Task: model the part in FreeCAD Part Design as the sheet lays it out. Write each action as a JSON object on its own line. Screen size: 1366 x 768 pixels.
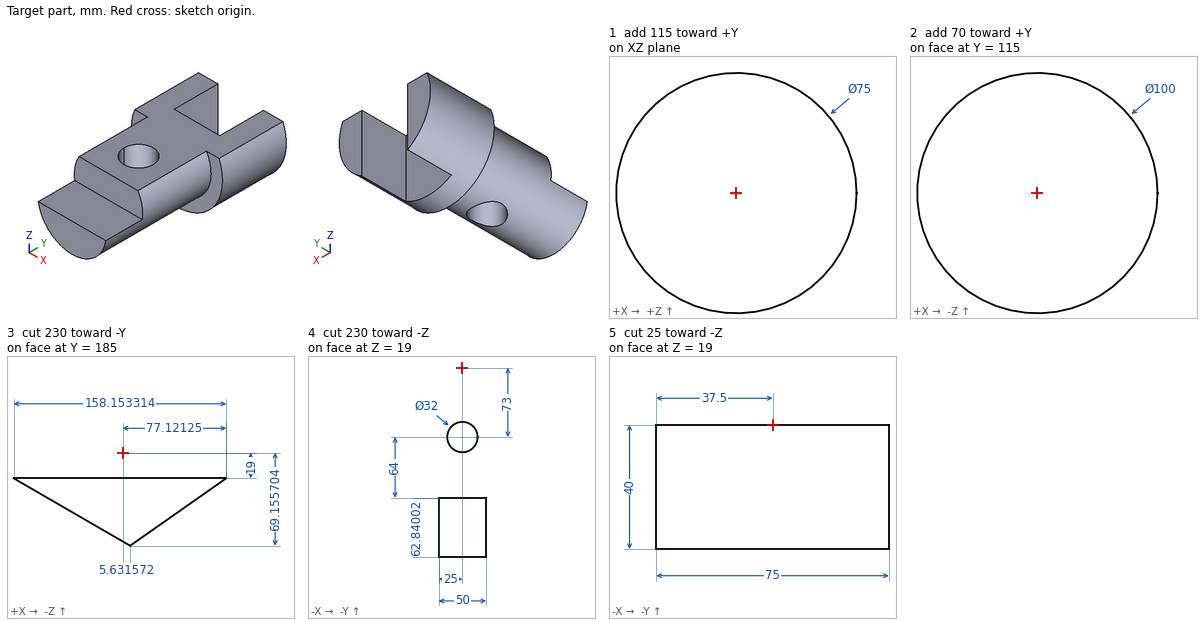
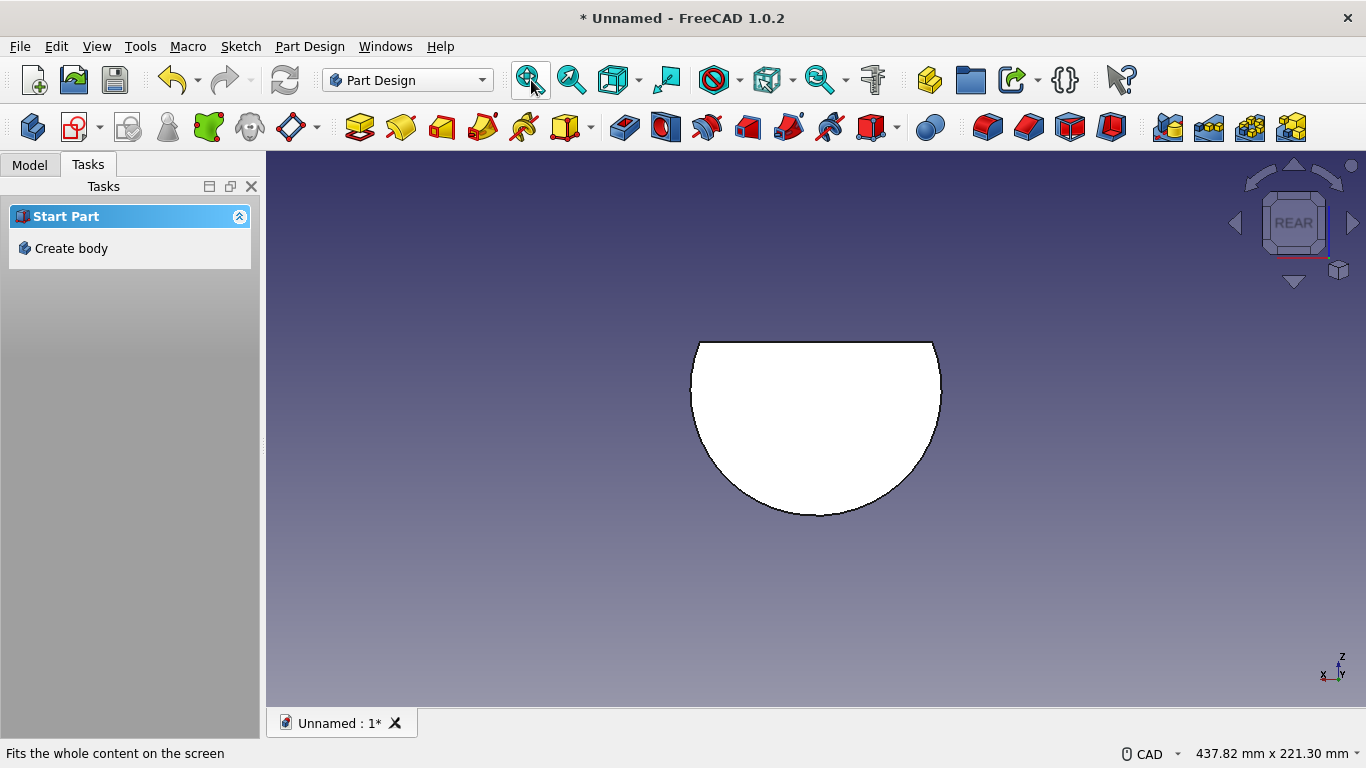
{"action": "key", "text": "0"}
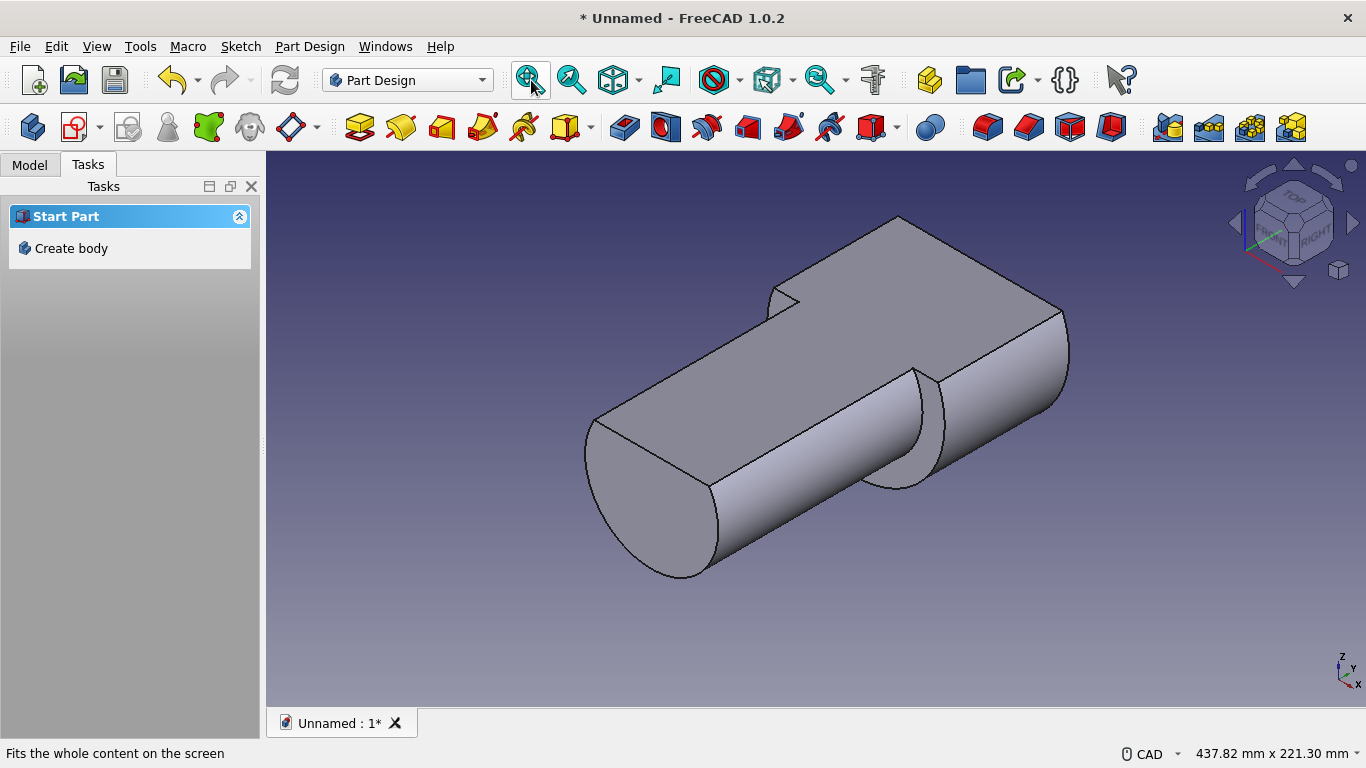
{"action": "left_click", "coordinate": [910, 303]}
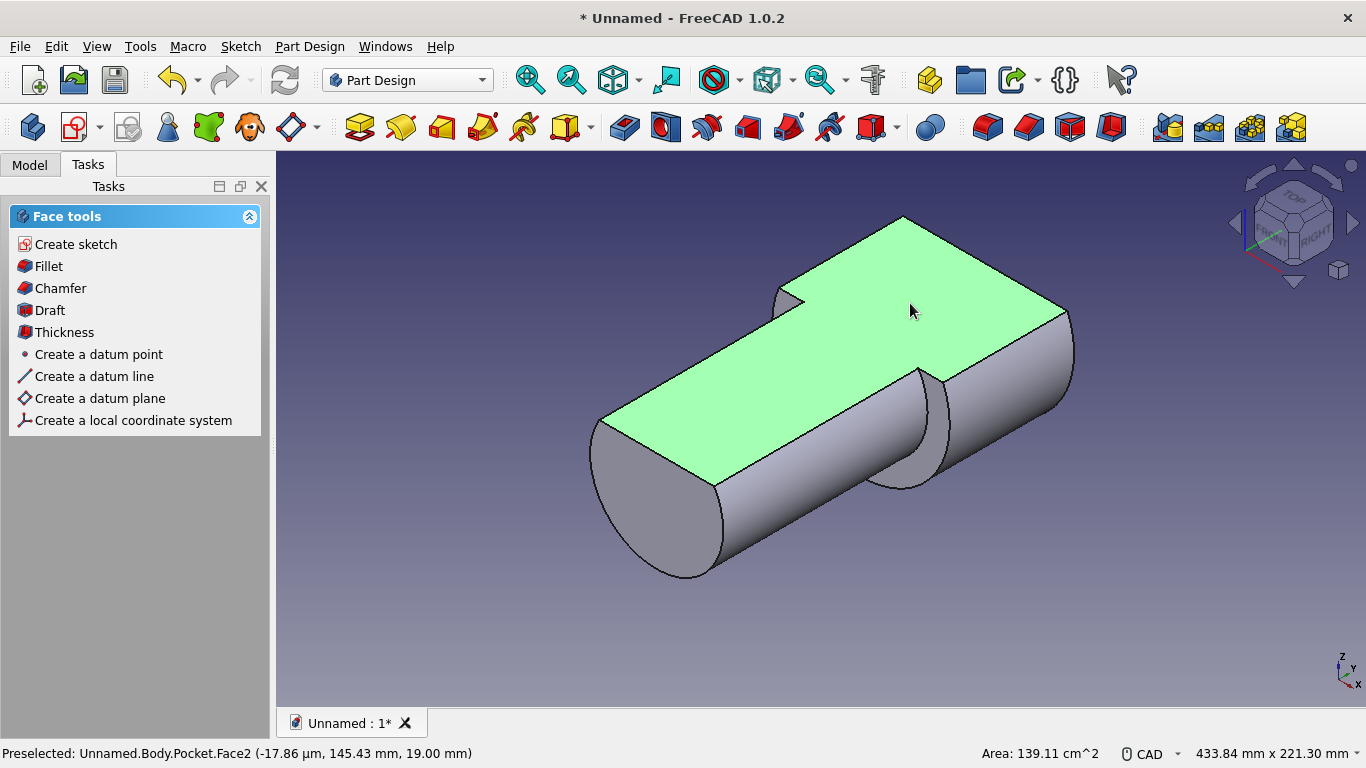
{"action": "left_click", "coordinate": [74, 128]}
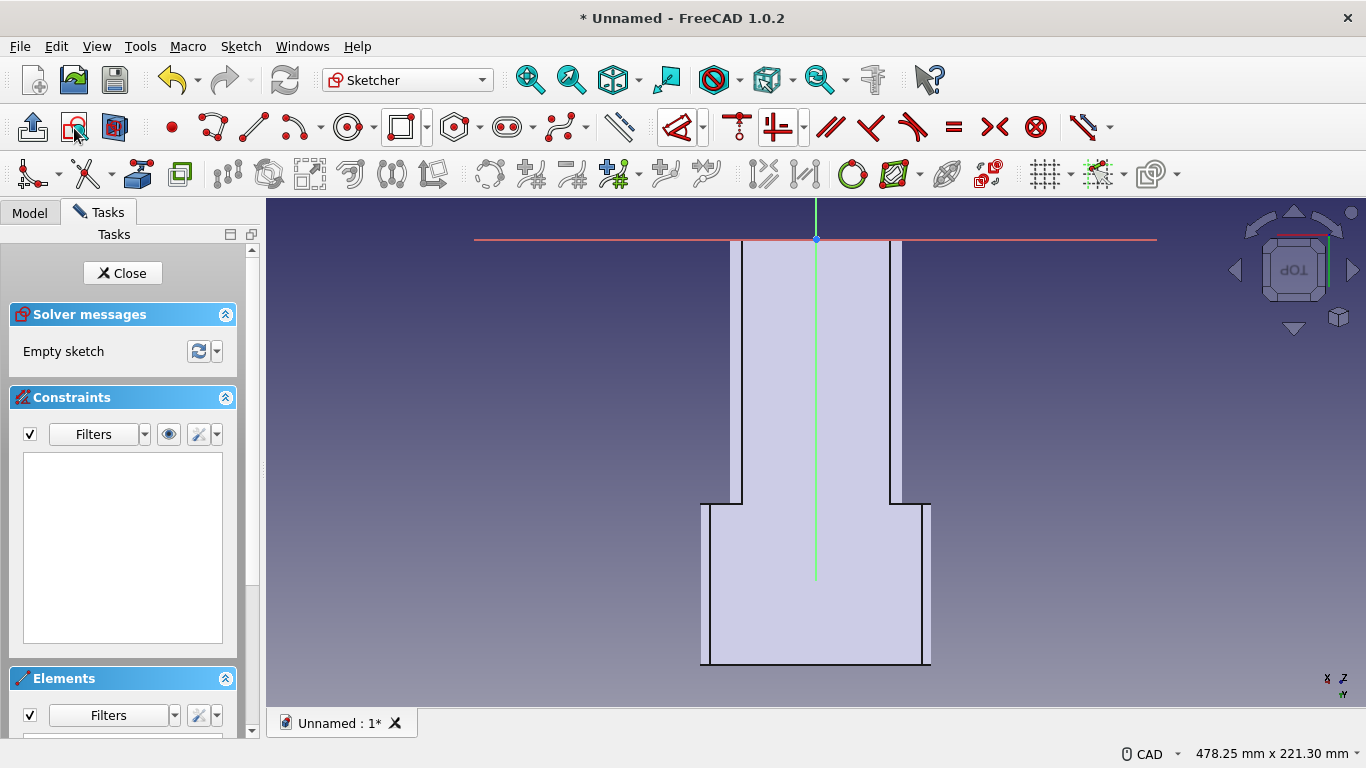
{"action": "scroll", "coordinate": [608, 418], "scroll_direction": "down", "scroll_amount": 2}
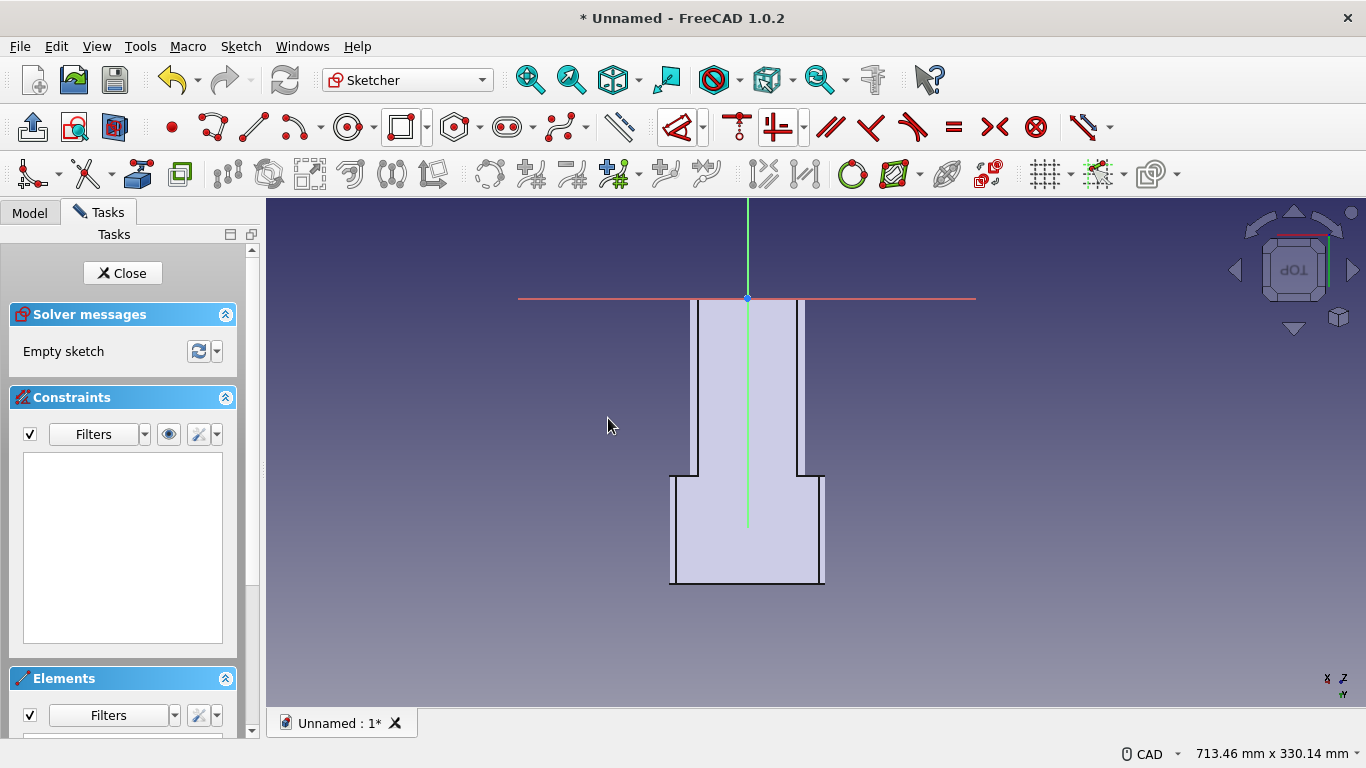
{"action": "left_click", "coordinate": [400, 128]}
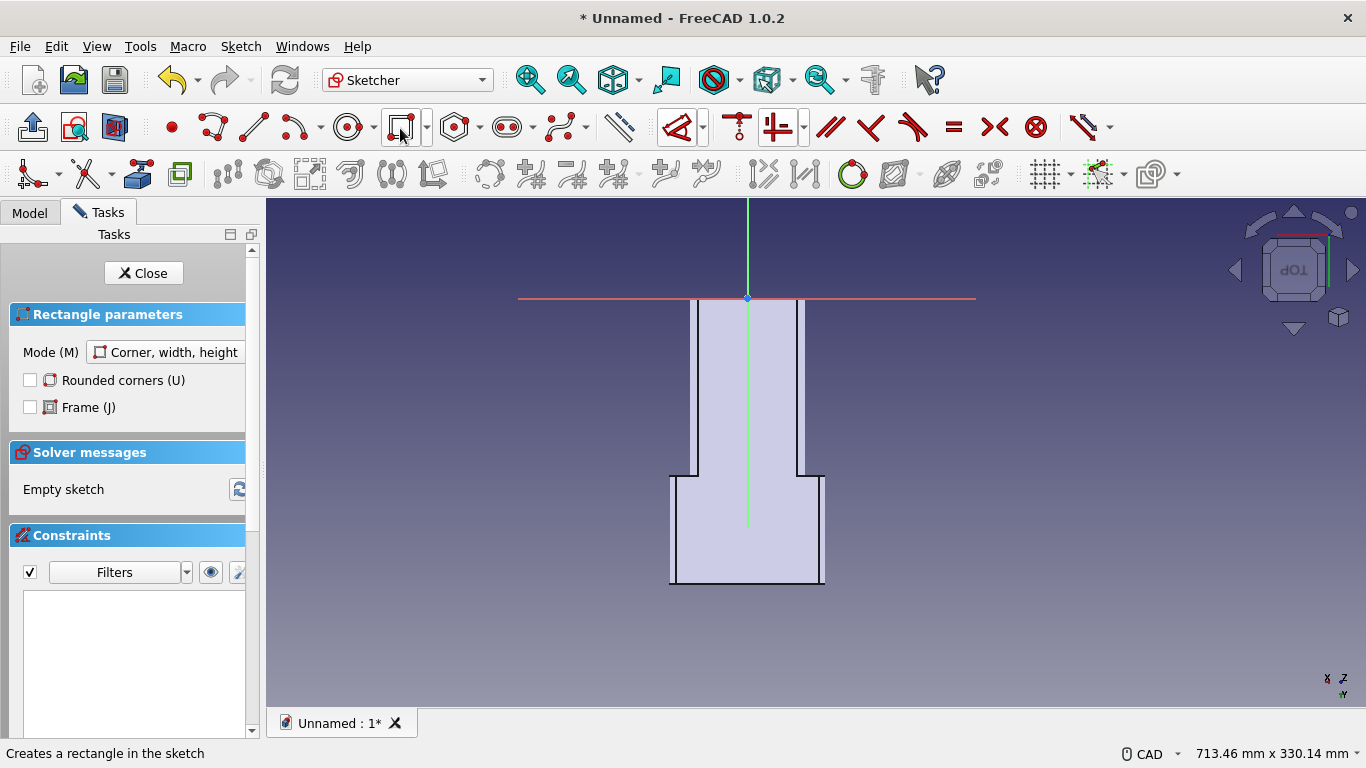
{"action": "left_click", "coordinate": [709, 510]}
{"action": "left_click", "coordinate": [786, 607]}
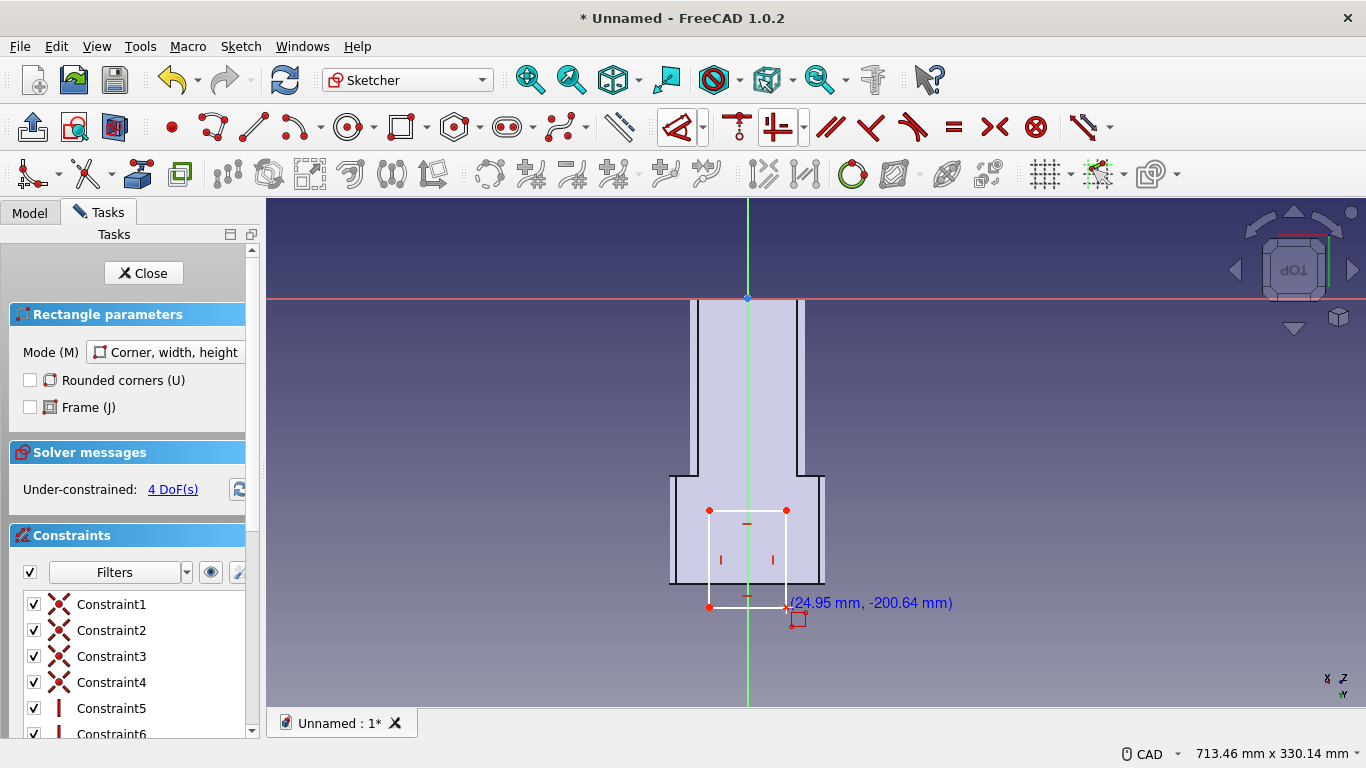
{"action": "left_click", "coordinate": [348, 128]}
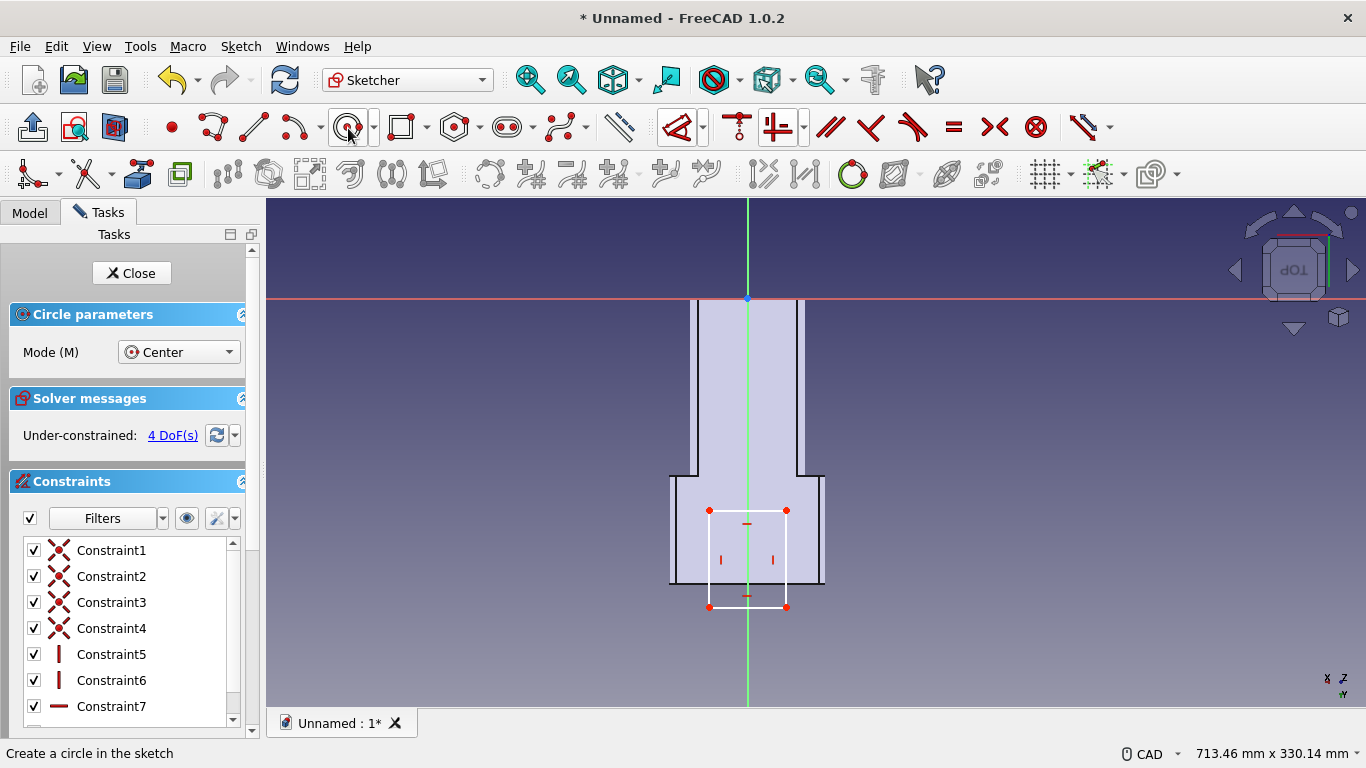
{"action": "left_click", "coordinate": [748, 411]}
{"action": "left_click", "coordinate": [765, 394]}
{"action": "key", "text": "Escape"}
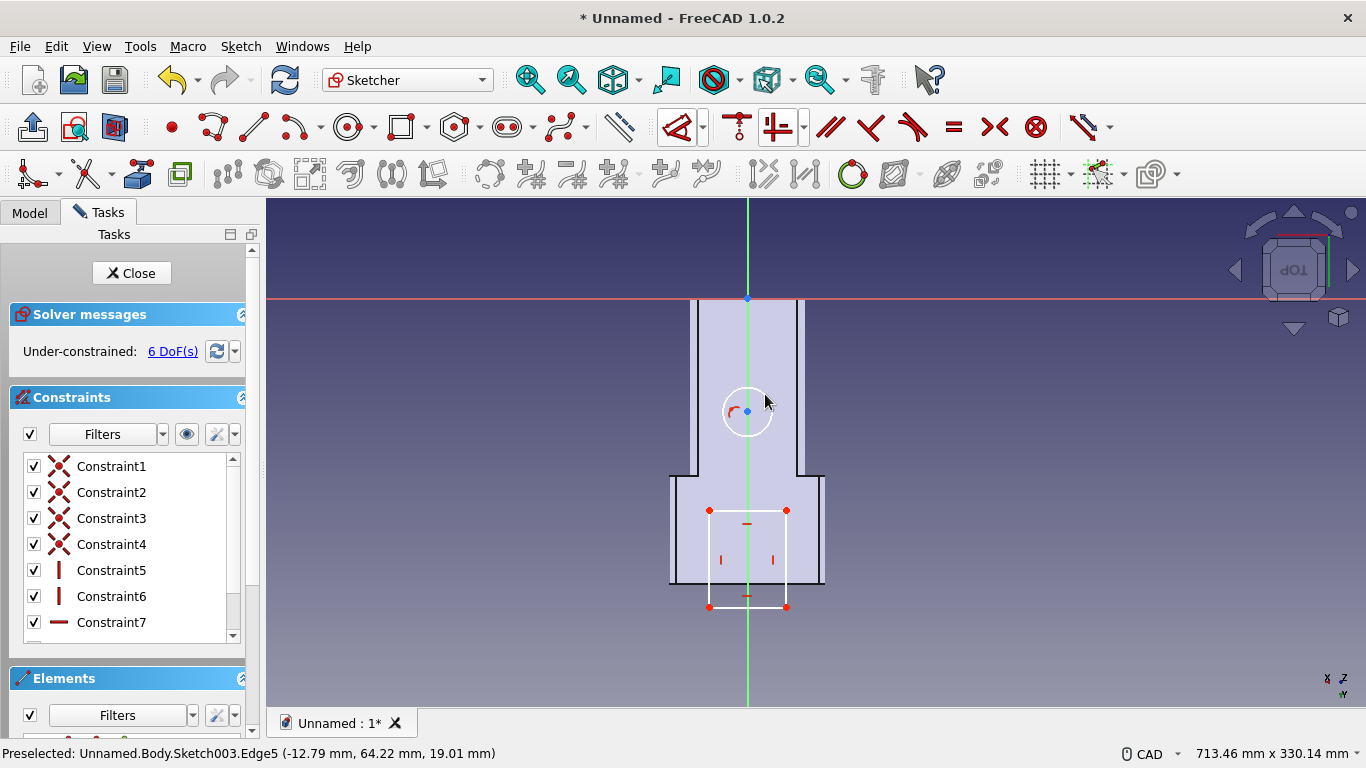
{"action": "left_click", "coordinate": [765, 395]}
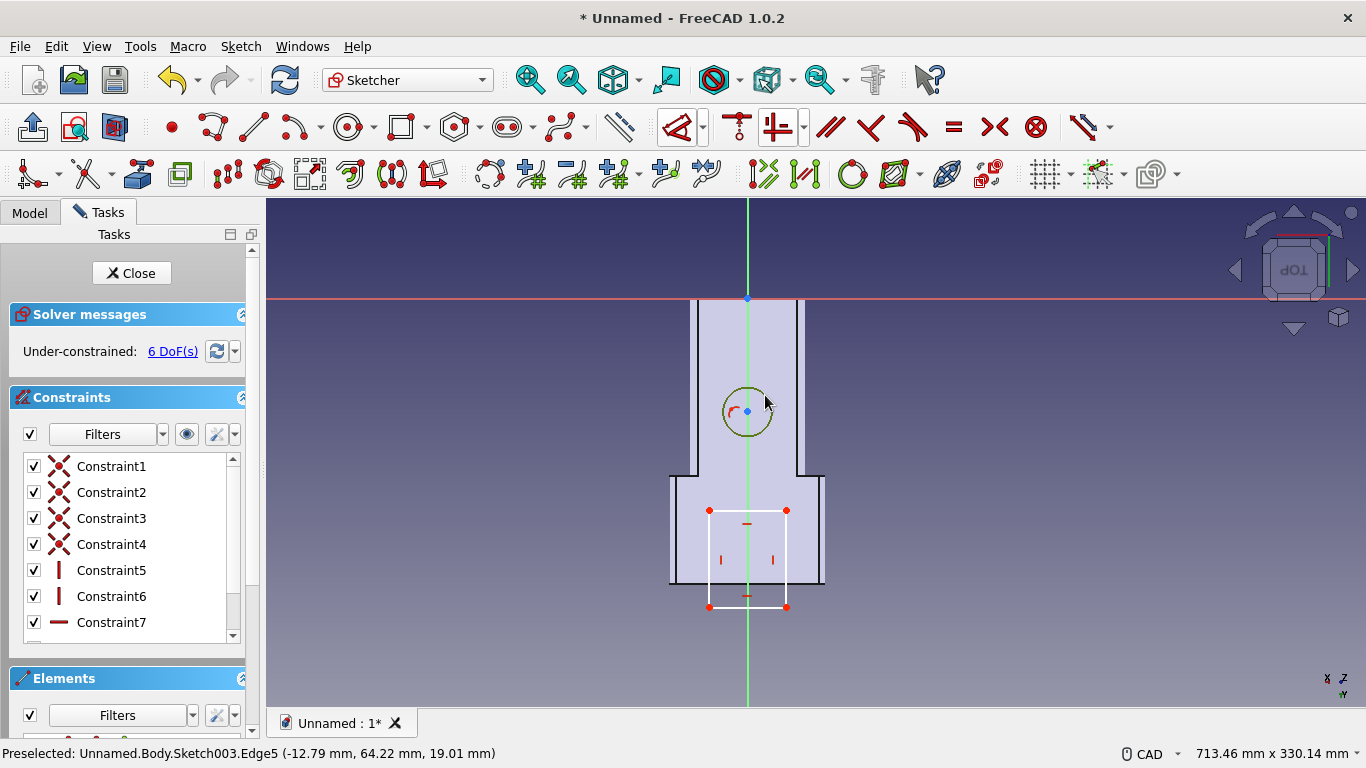
{"action": "left_click", "coordinate": [702, 128]}